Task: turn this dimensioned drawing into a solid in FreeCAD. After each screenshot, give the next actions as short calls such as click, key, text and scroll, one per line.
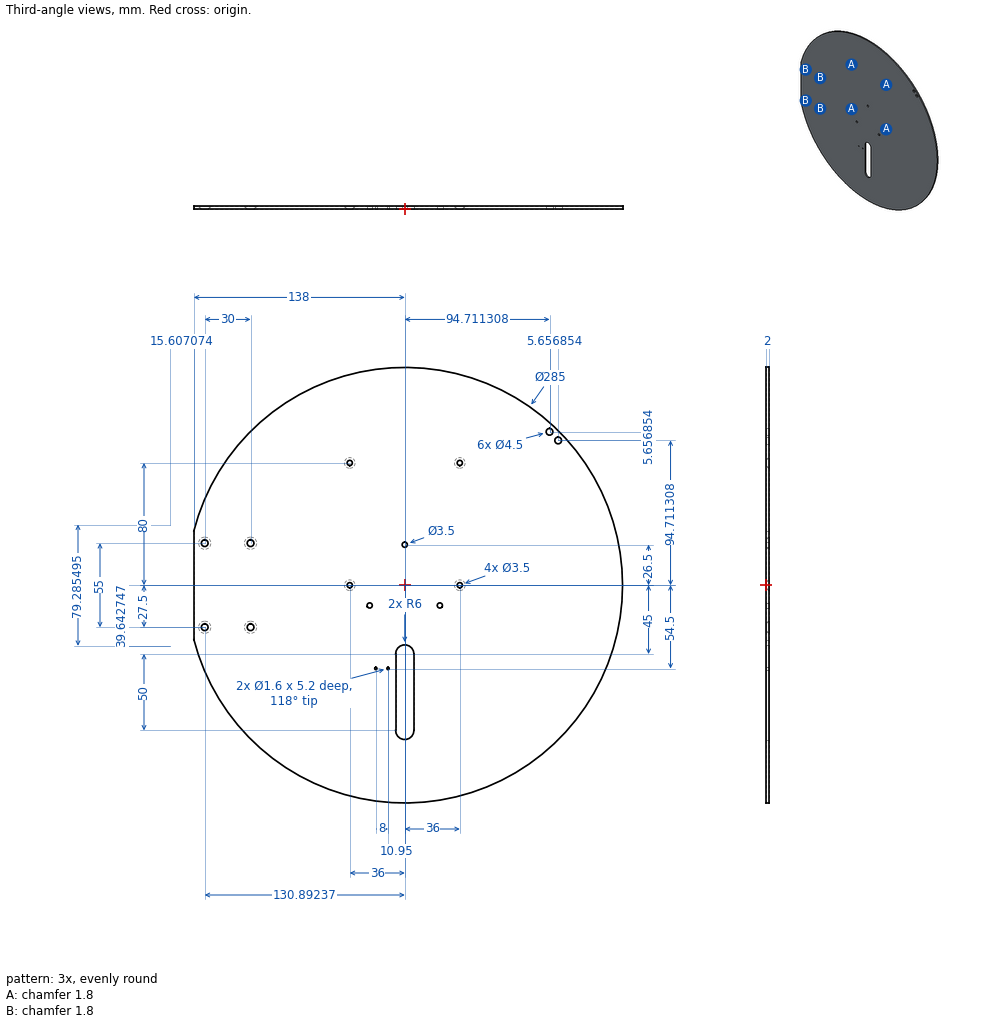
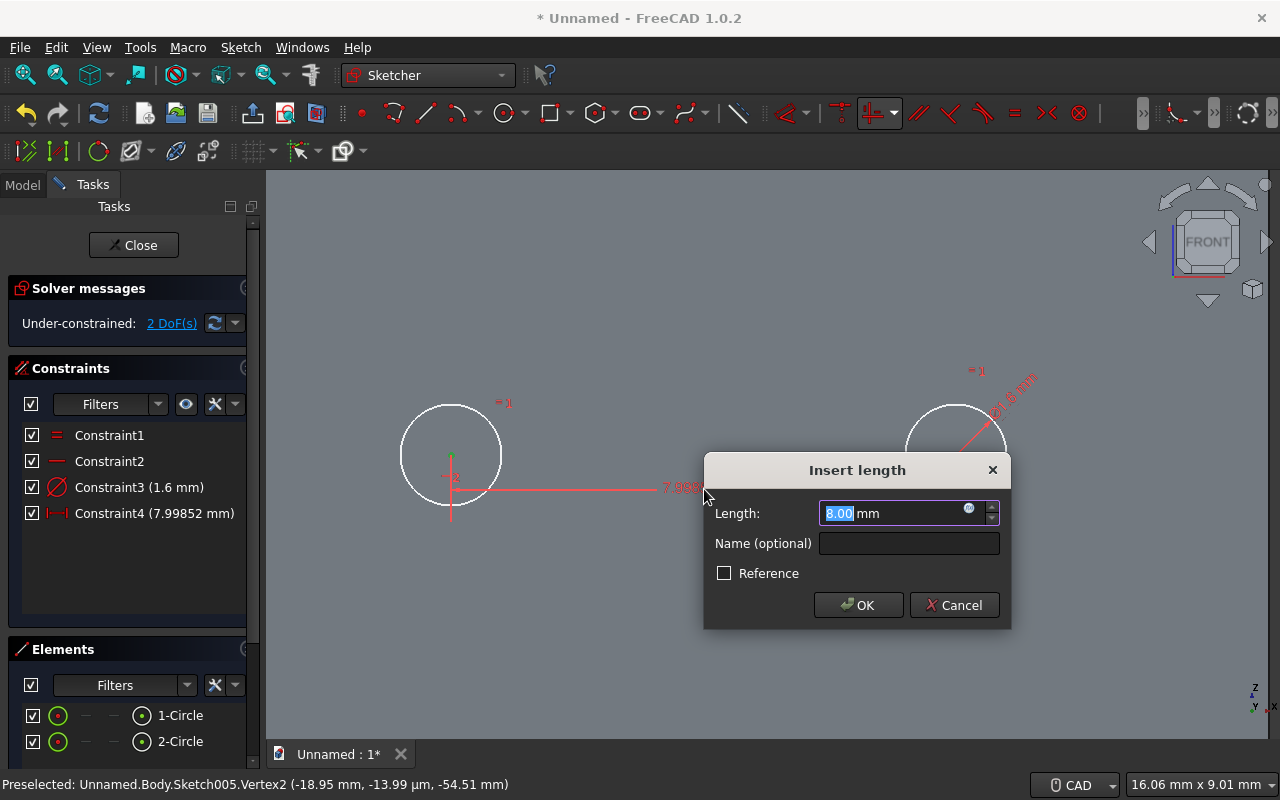
text(8)
key(Return)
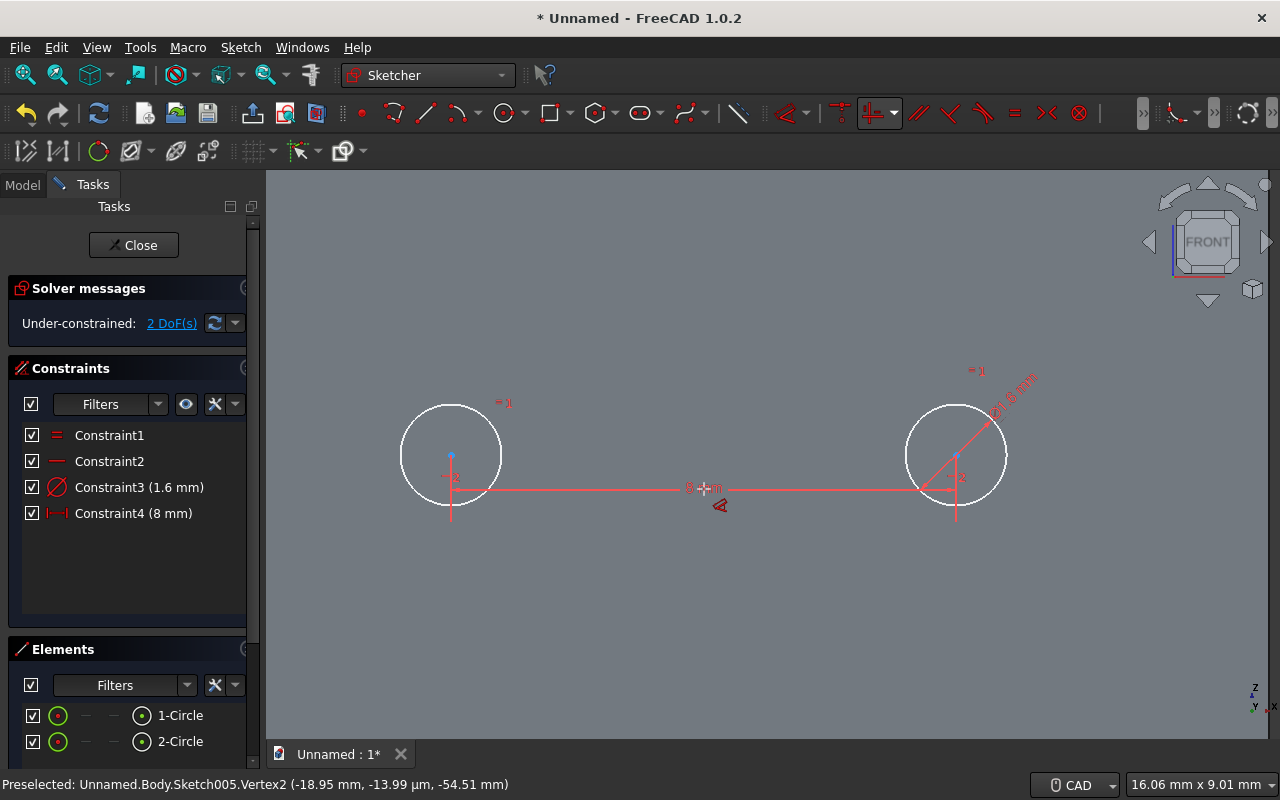
click(956, 455)
click(922, 326)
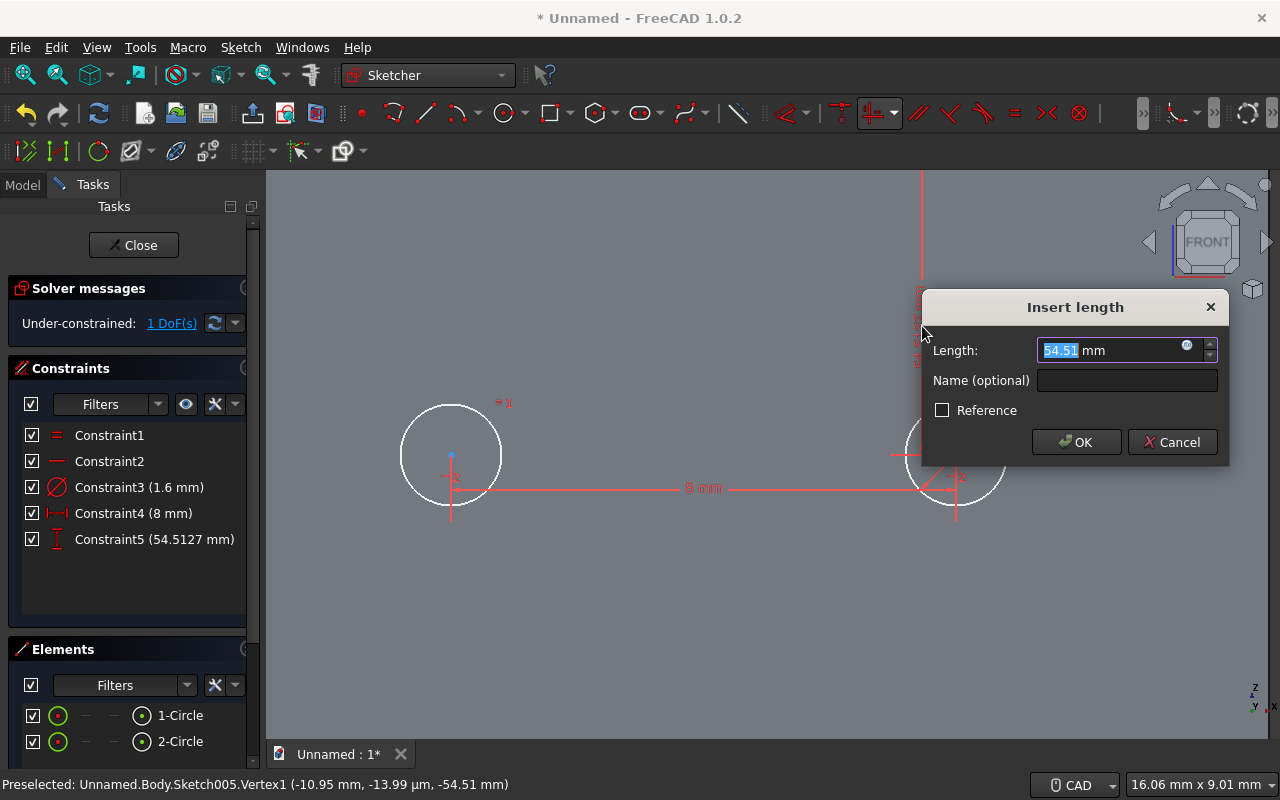
text(54.5)
key(Return)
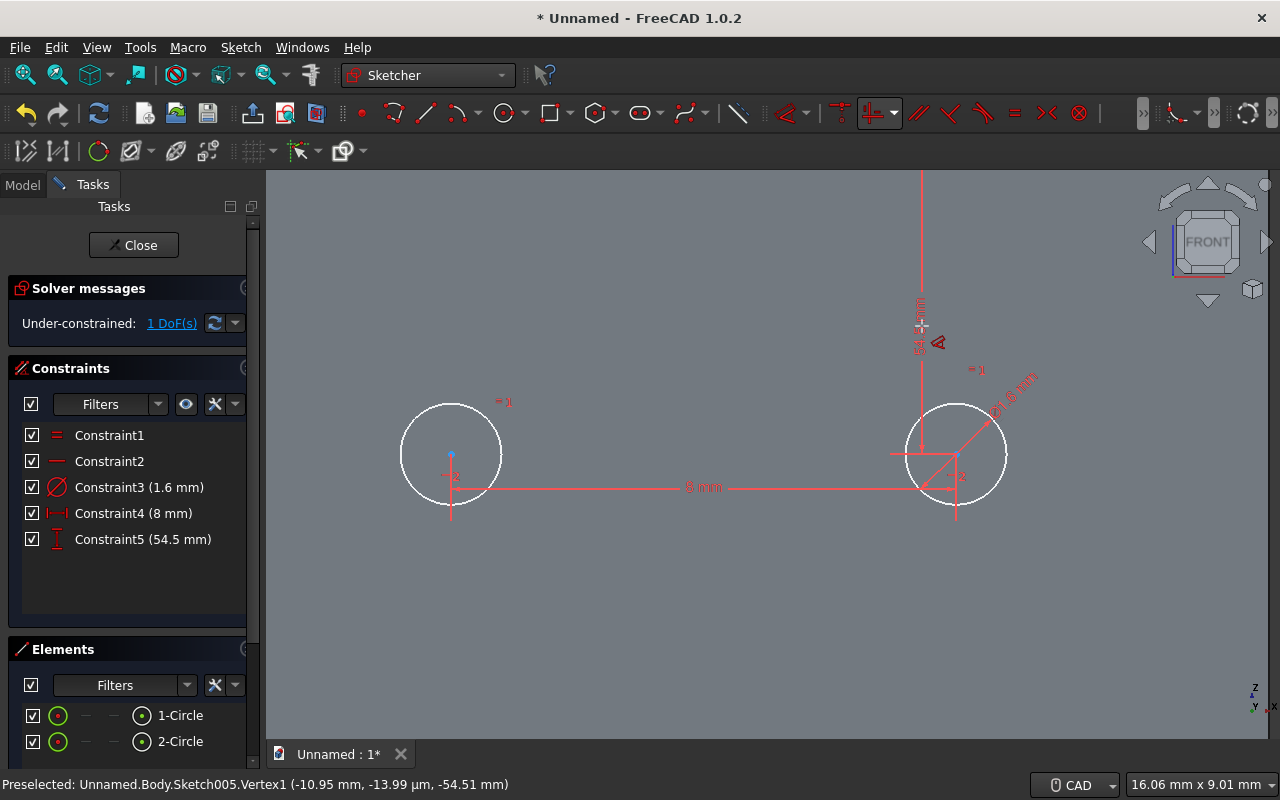
click(956, 454)
click(1036, 488)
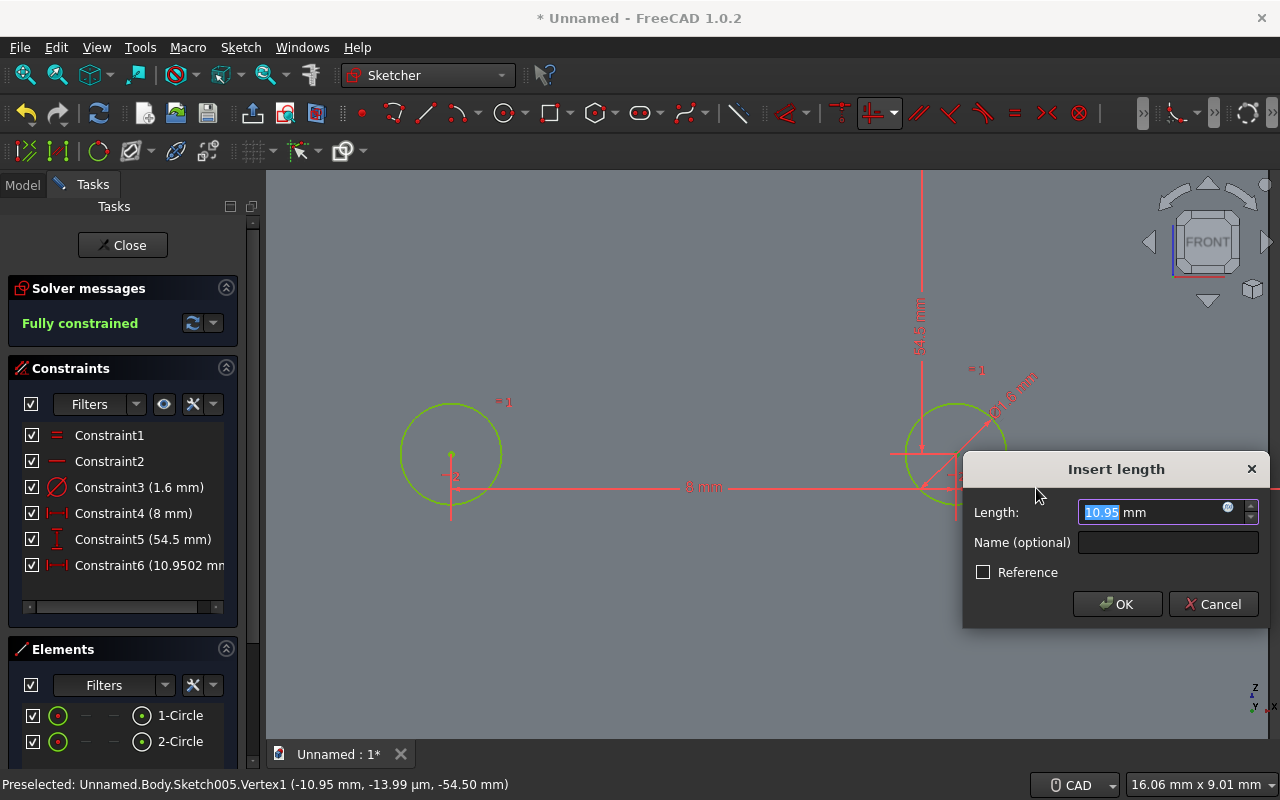
text(10.95)
key(Return)
key(Escape)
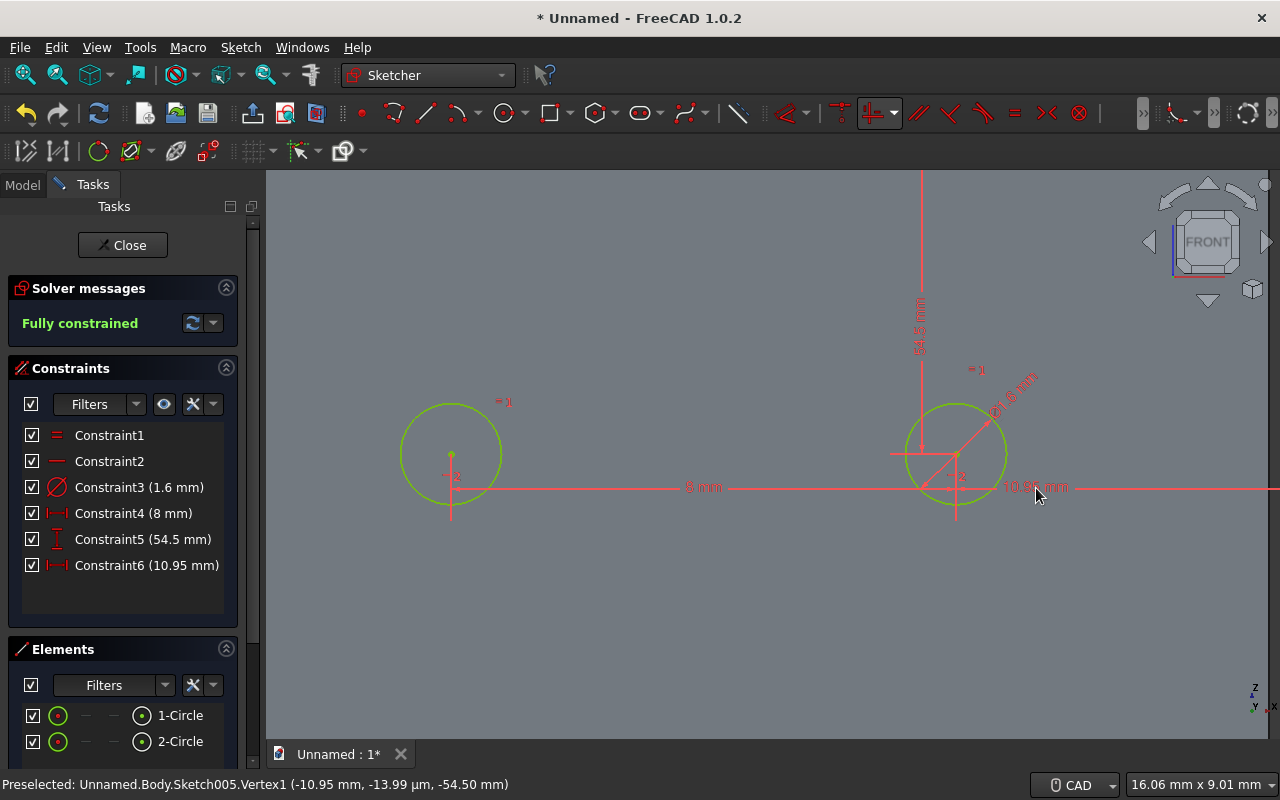
click(123, 245)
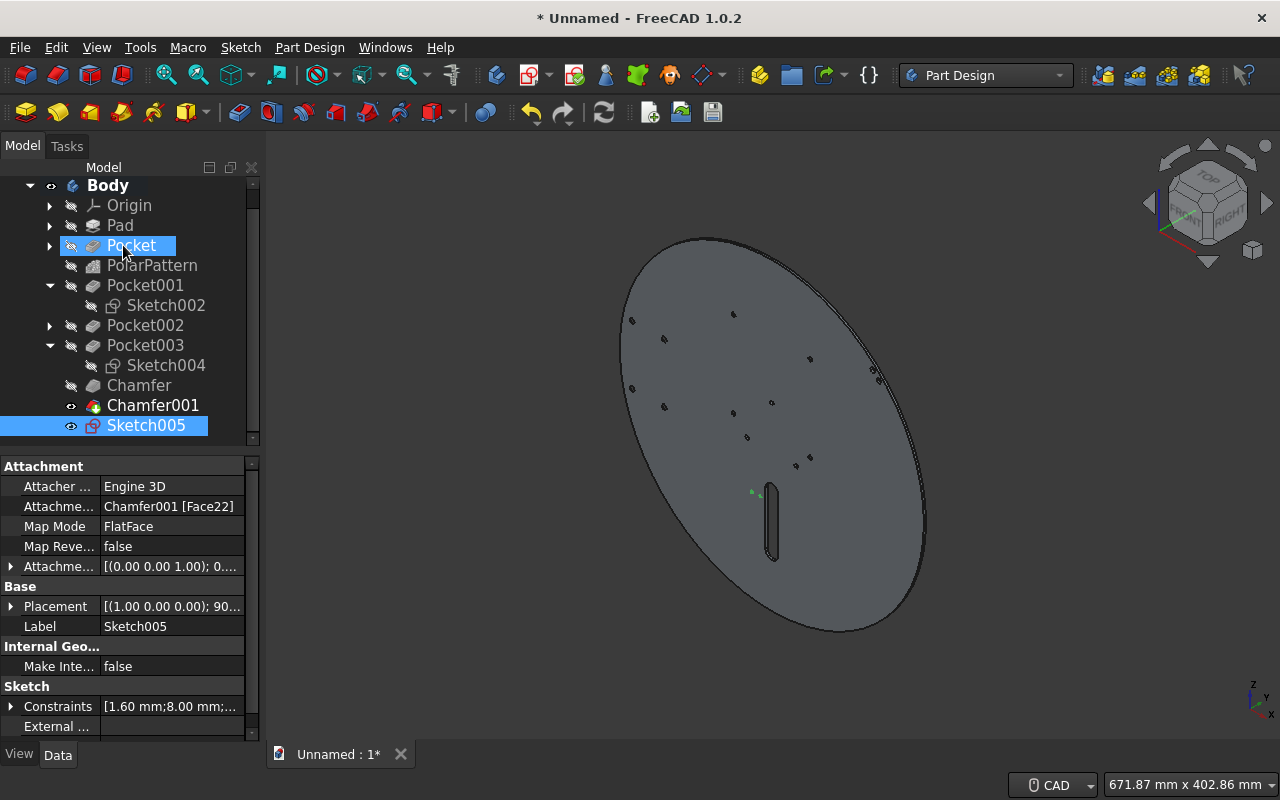
click(272, 112)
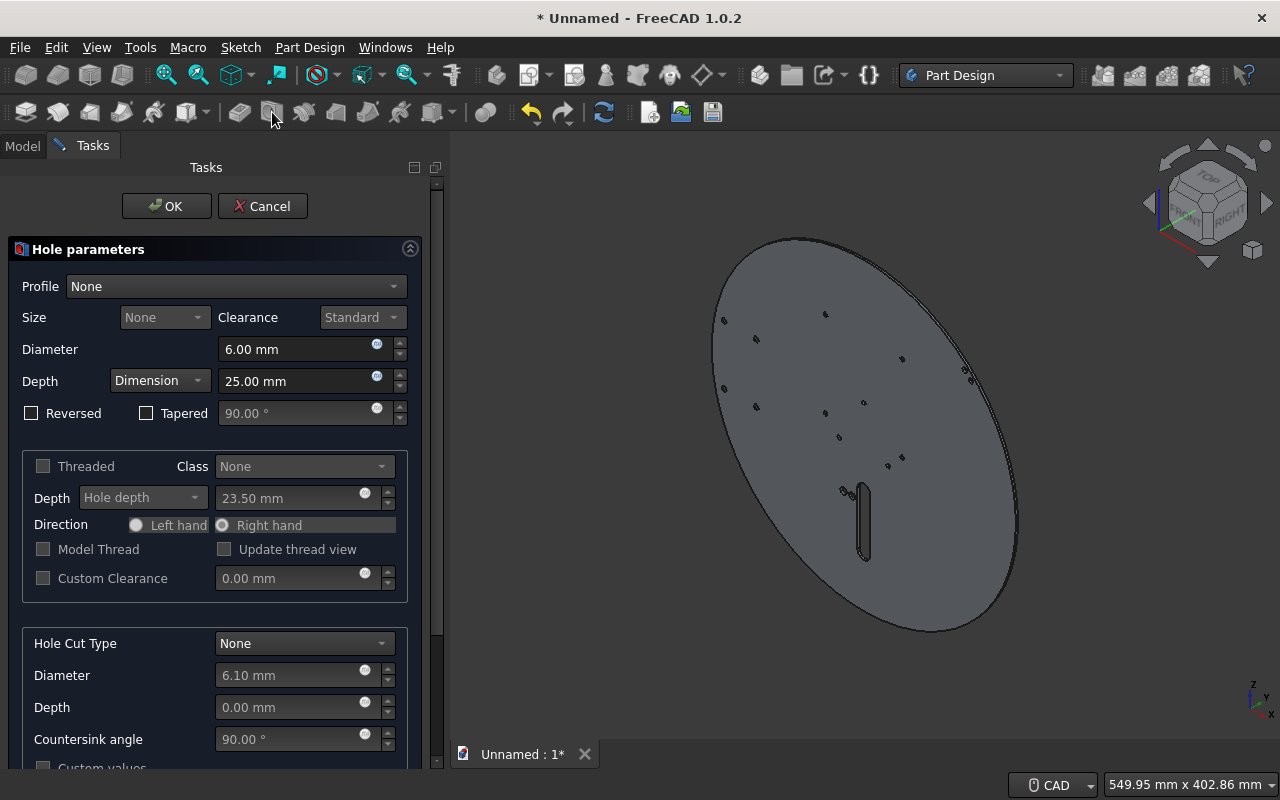
triple_click(305, 349)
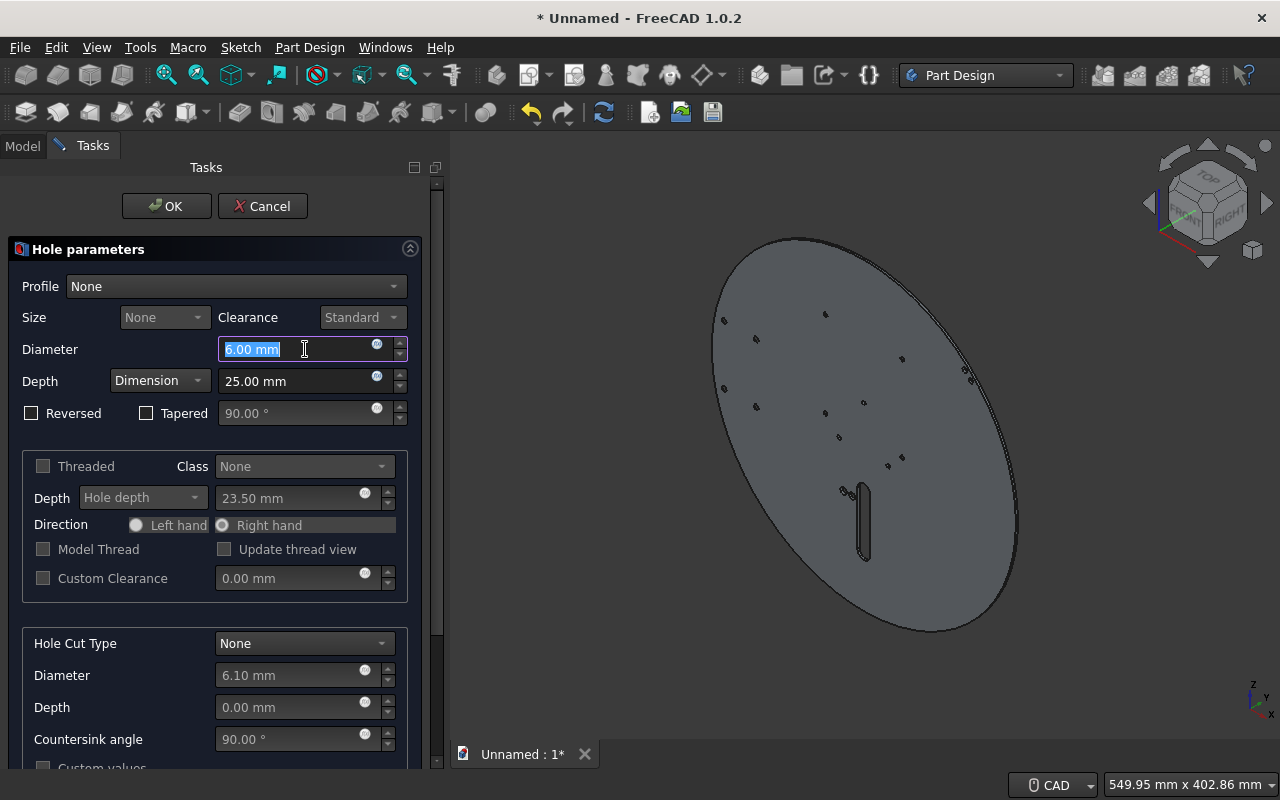
text(1.6)
key(Tab)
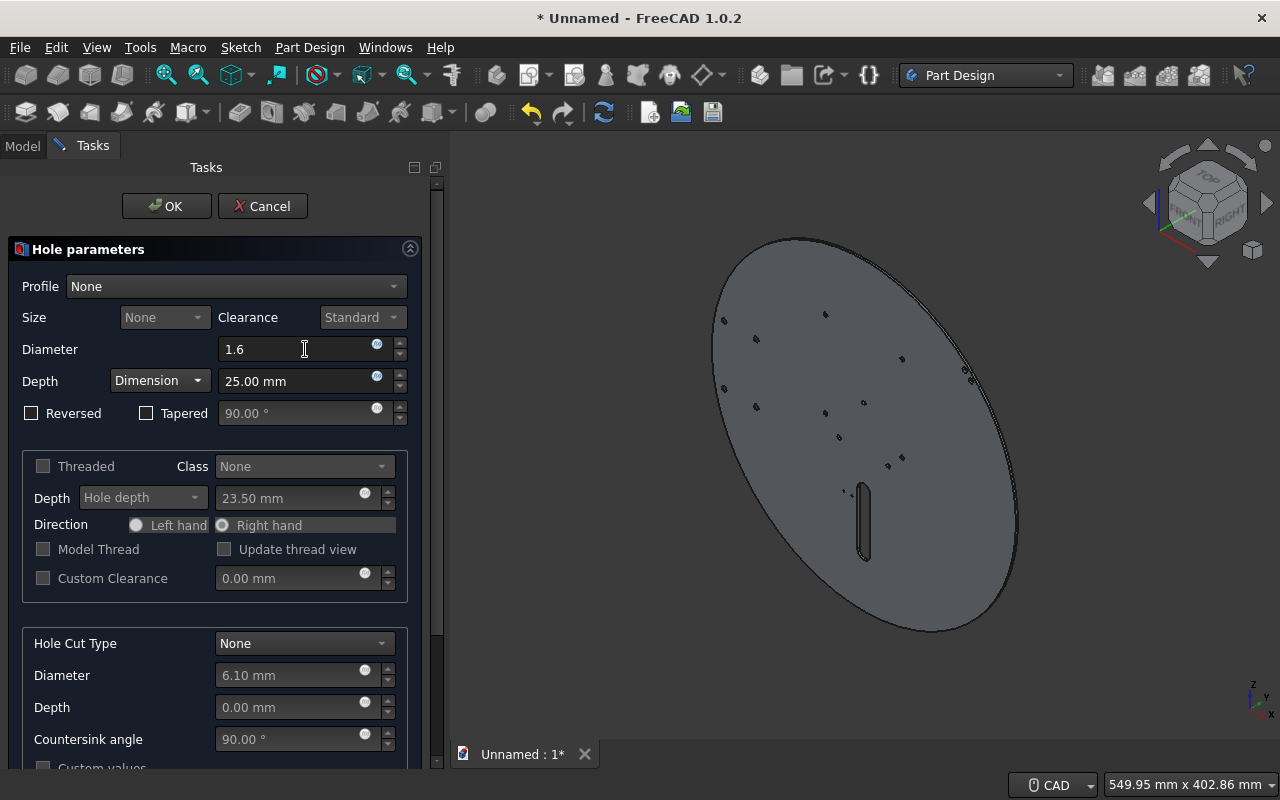
triple_click(305, 381)